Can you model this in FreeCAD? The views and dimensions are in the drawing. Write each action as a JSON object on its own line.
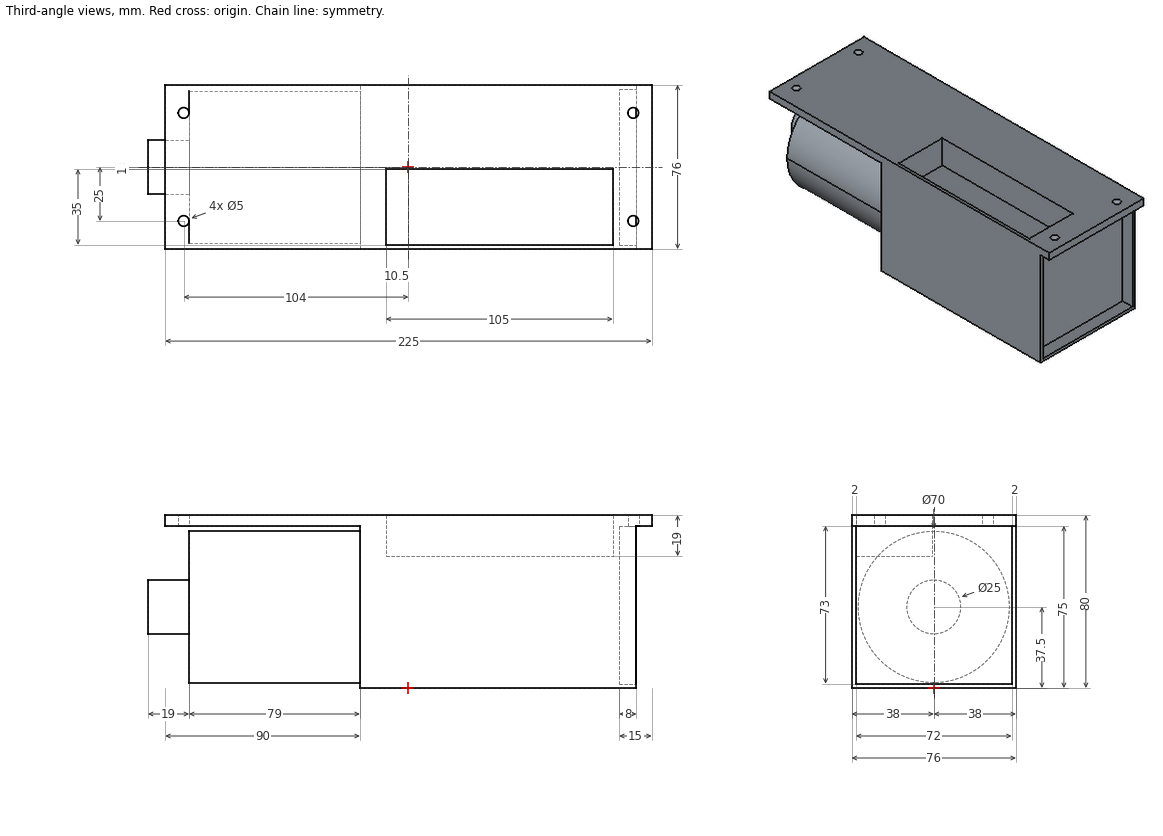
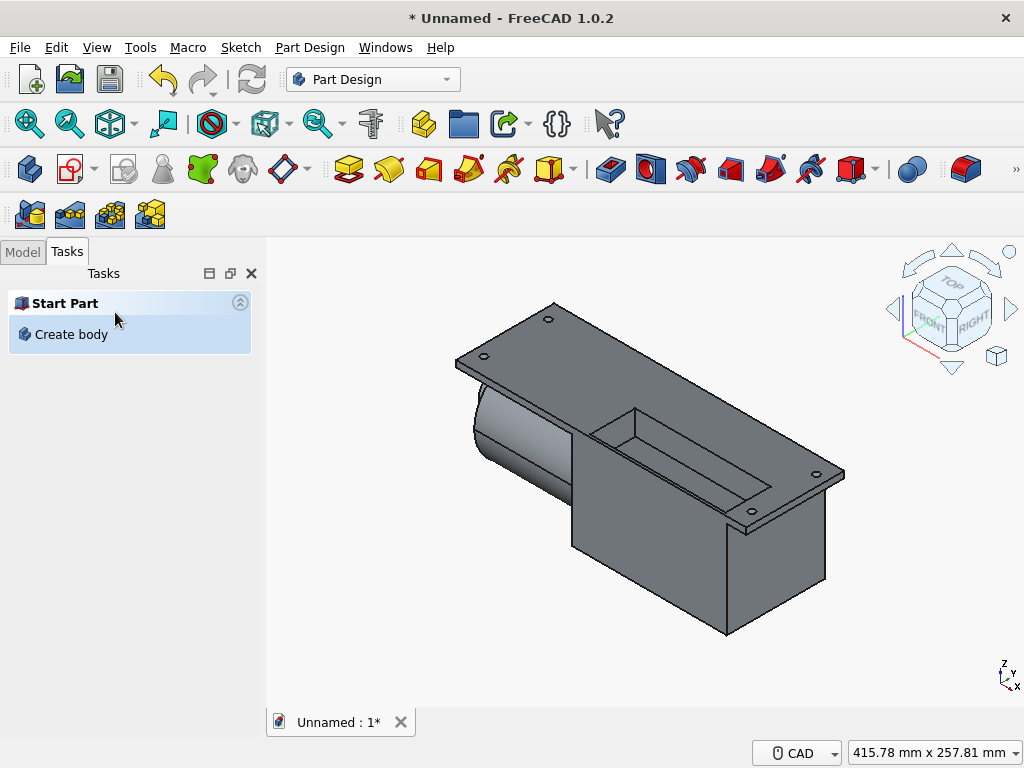
{"action": "left_click", "coordinate": [776, 550]}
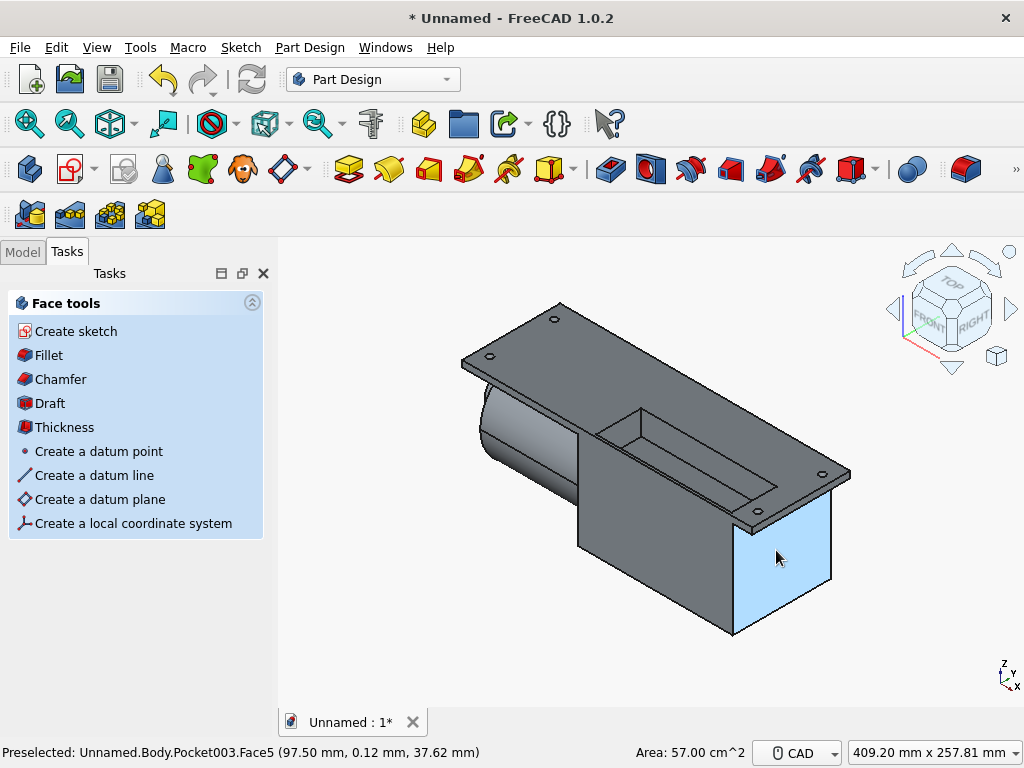
{"action": "left_click", "coordinate": [70, 170]}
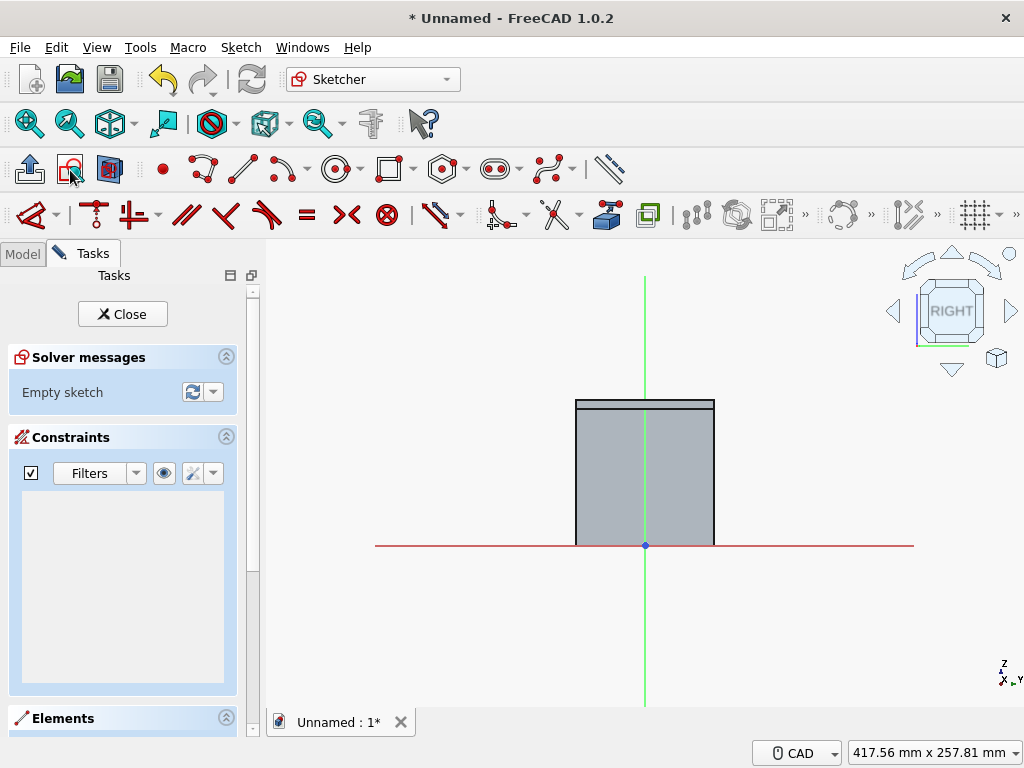
{"action": "scroll", "coordinate": [701, 481], "scroll_direction": "up", "scroll_amount": 4}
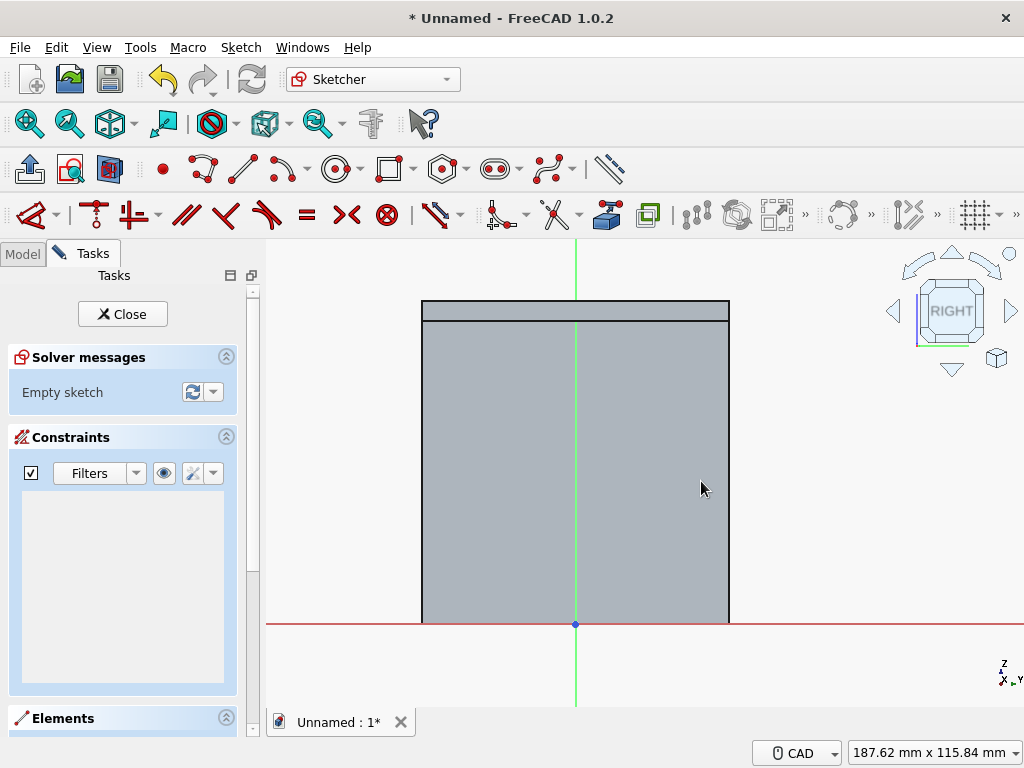
{"action": "key", "text": "g m"}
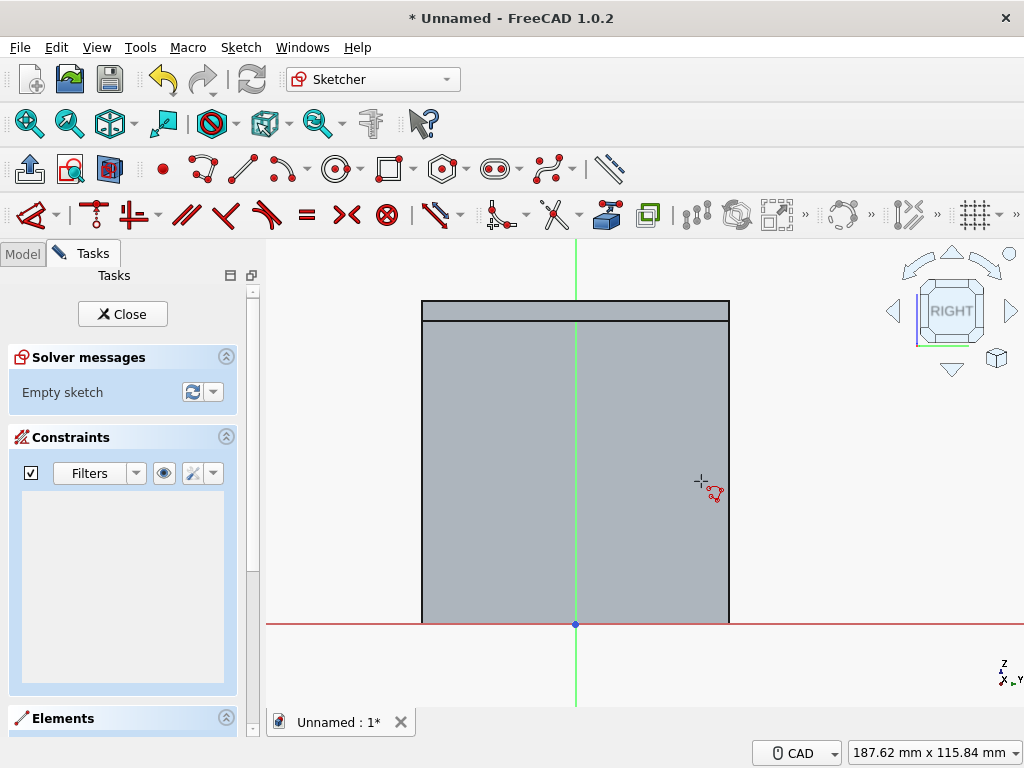
{"action": "scroll", "coordinate": [721, 616], "scroll_direction": "up", "scroll_amount": 4}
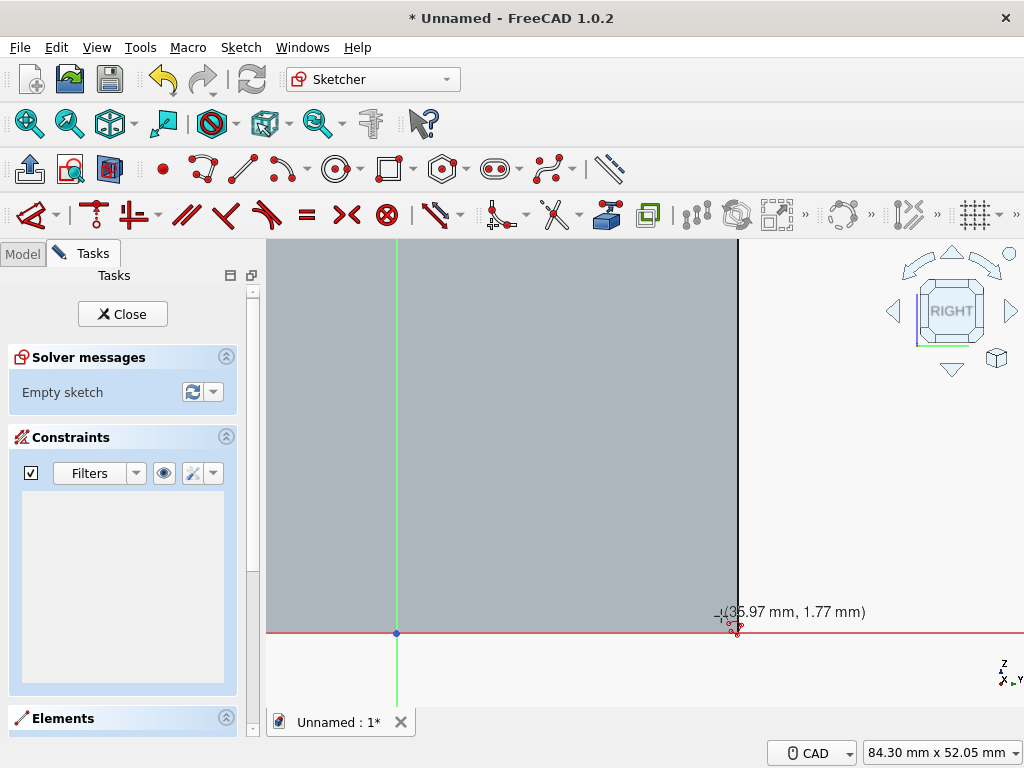
{"action": "left_click", "coordinate": [721, 615]}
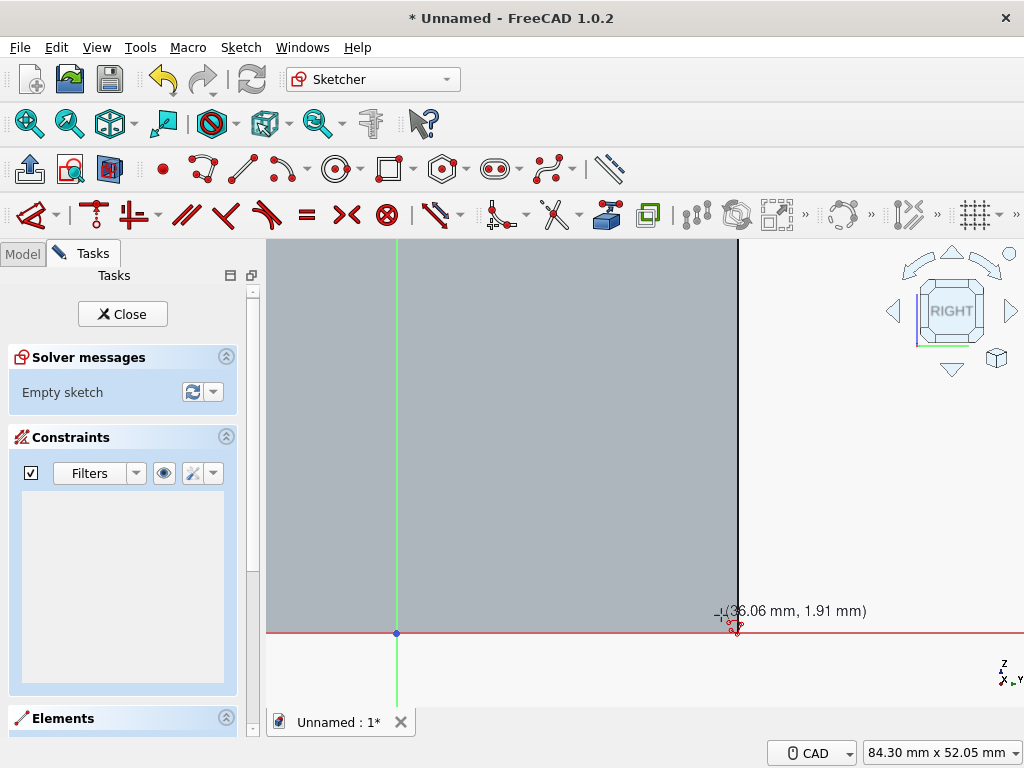
{"action": "scroll", "coordinate": [723, 617], "scroll_direction": "down", "scroll_amount": 4}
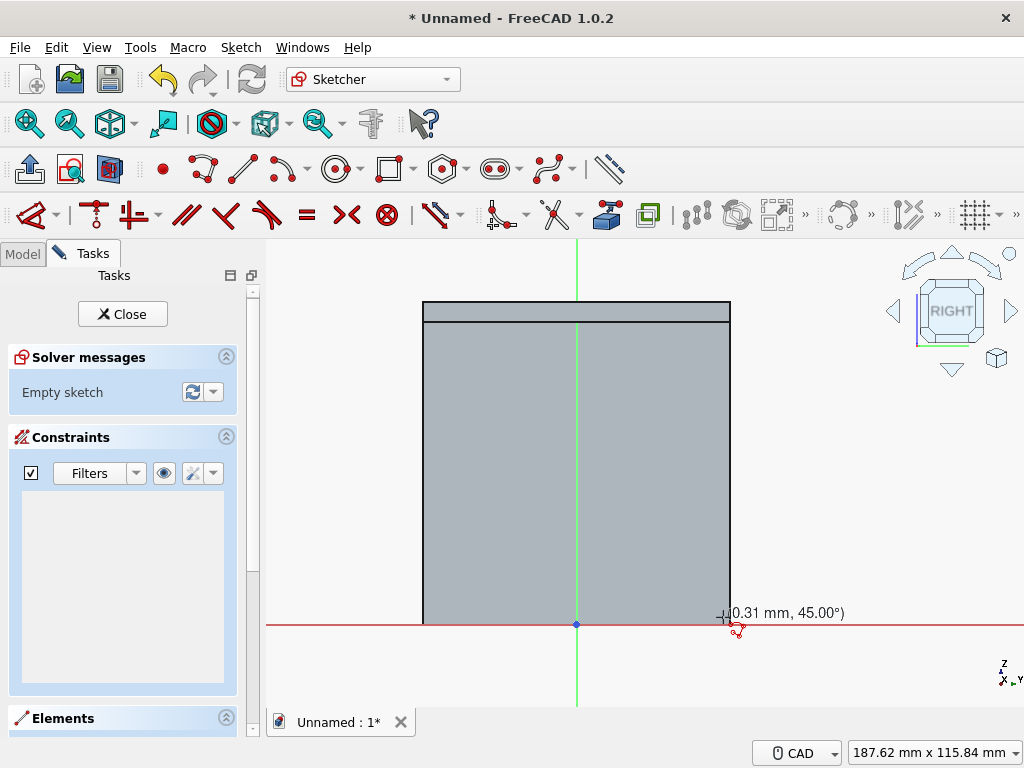
{"action": "scroll", "coordinate": [431, 617], "scroll_direction": "up", "scroll_amount": 4}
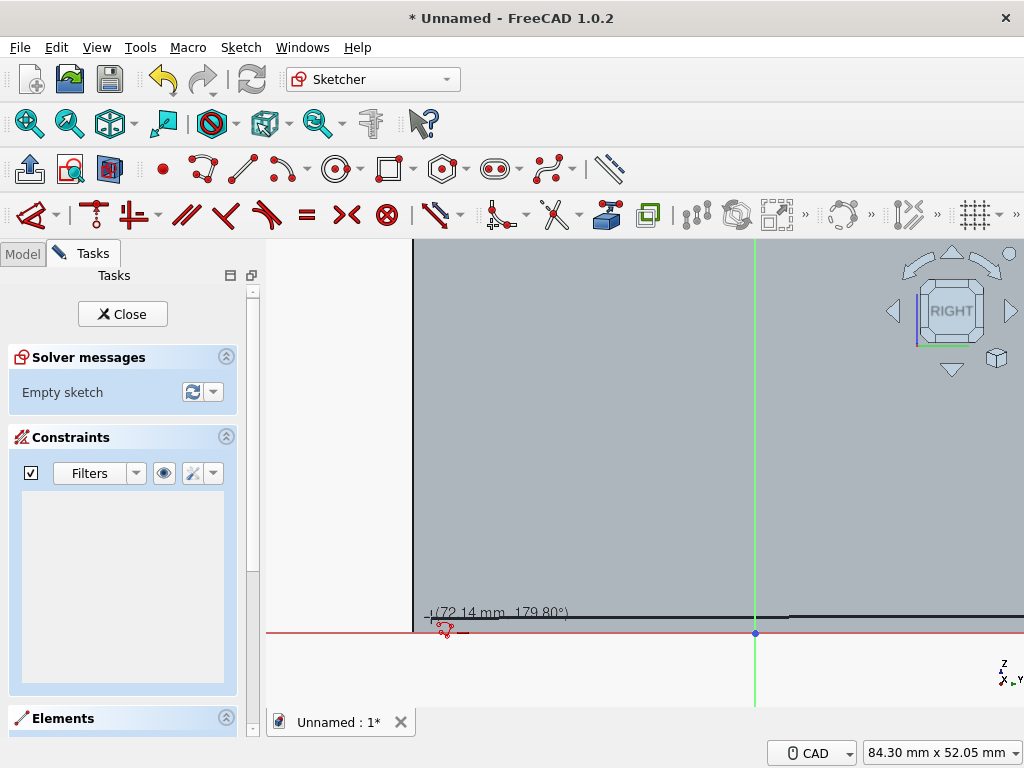
{"action": "left_click", "coordinate": [431, 615]}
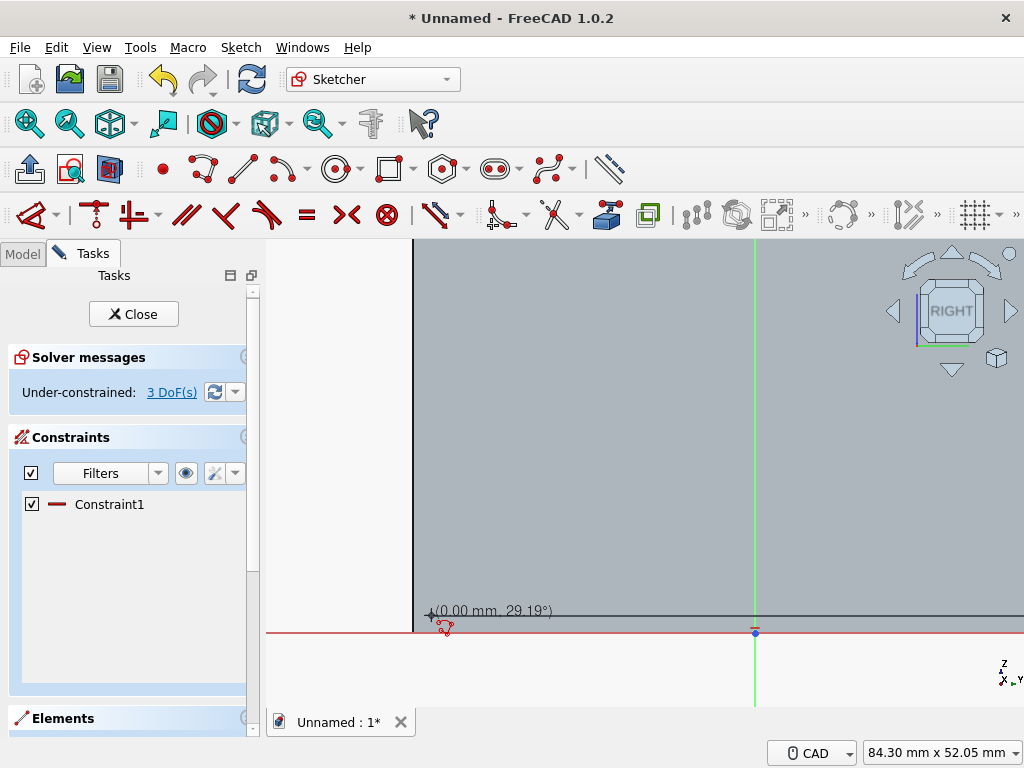
{"action": "scroll", "coordinate": [431, 617], "scroll_direction": "down", "scroll_amount": 4}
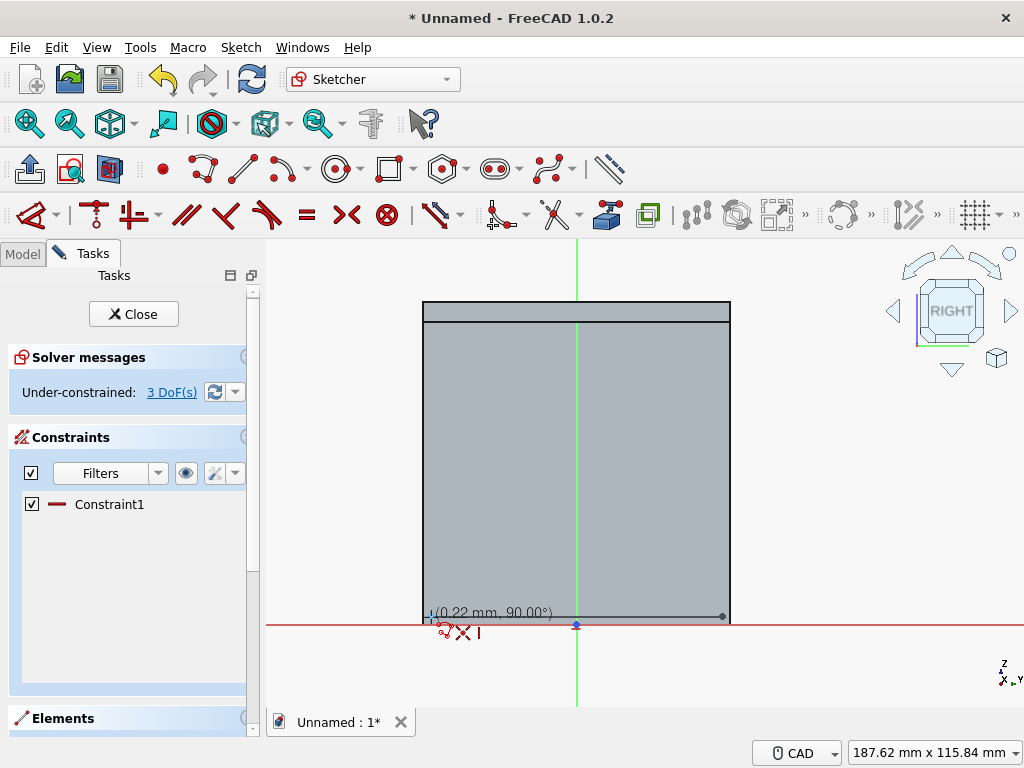
{"action": "left_click", "coordinate": [431, 322]}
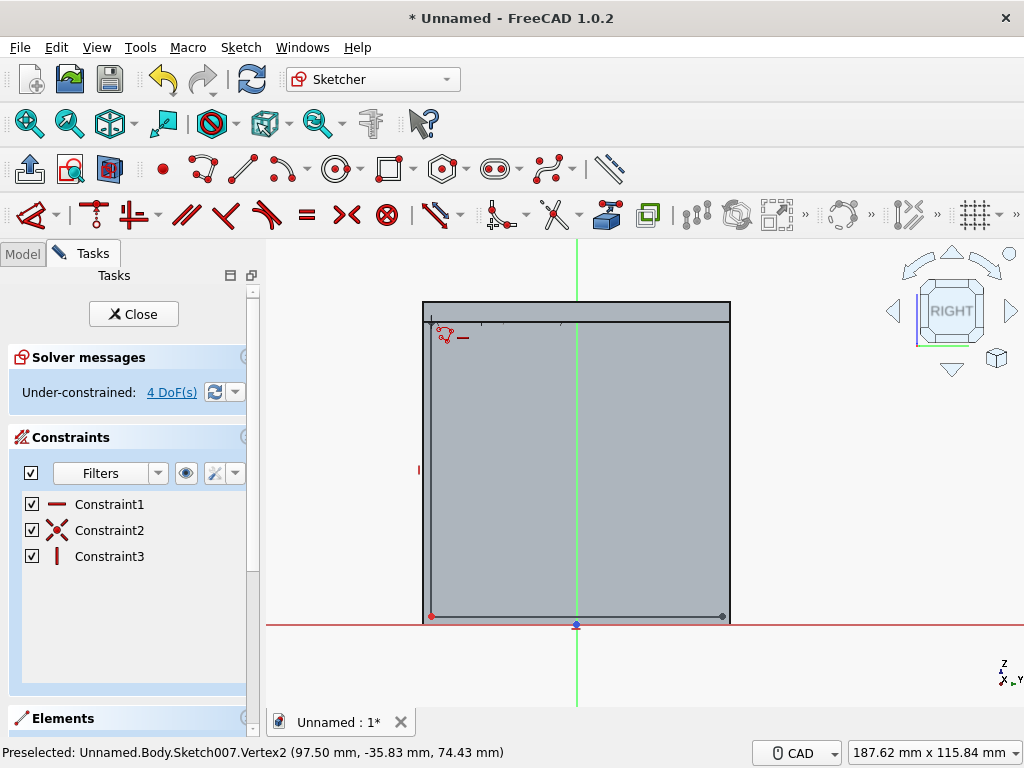
{"action": "scroll", "coordinate": [423, 322], "scroll_direction": "up", "scroll_amount": 4}